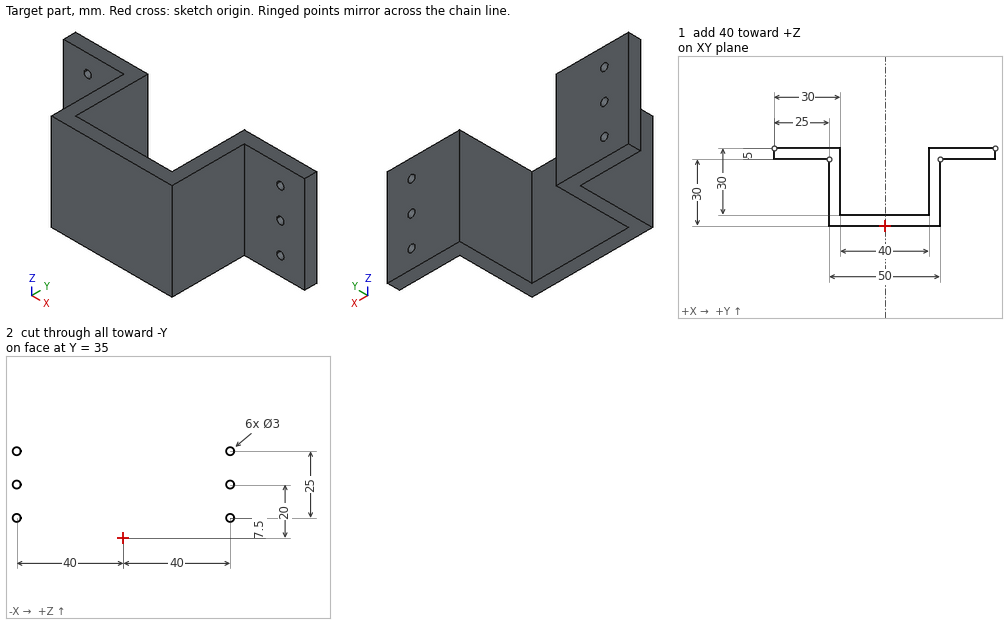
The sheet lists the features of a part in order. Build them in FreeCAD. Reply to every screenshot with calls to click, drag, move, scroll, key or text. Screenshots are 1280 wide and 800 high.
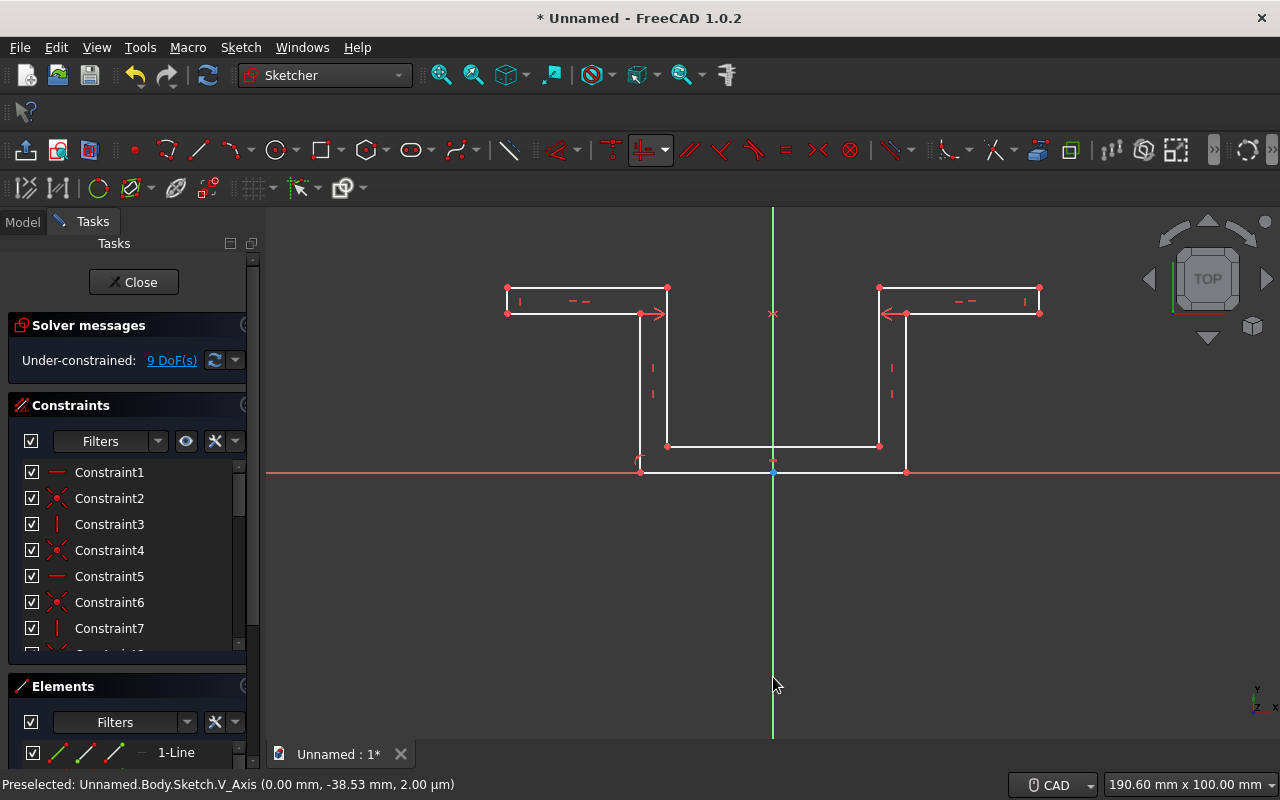
click(507, 288)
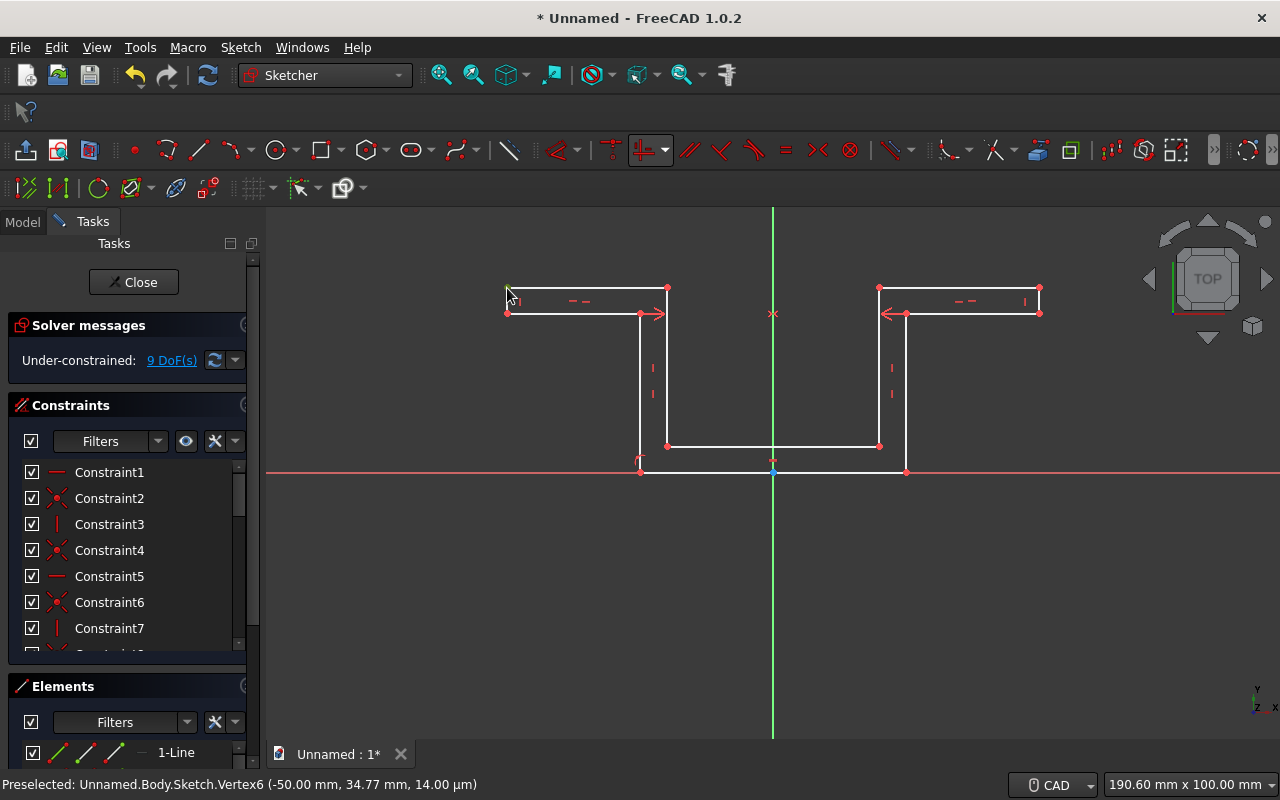
click(1039, 288)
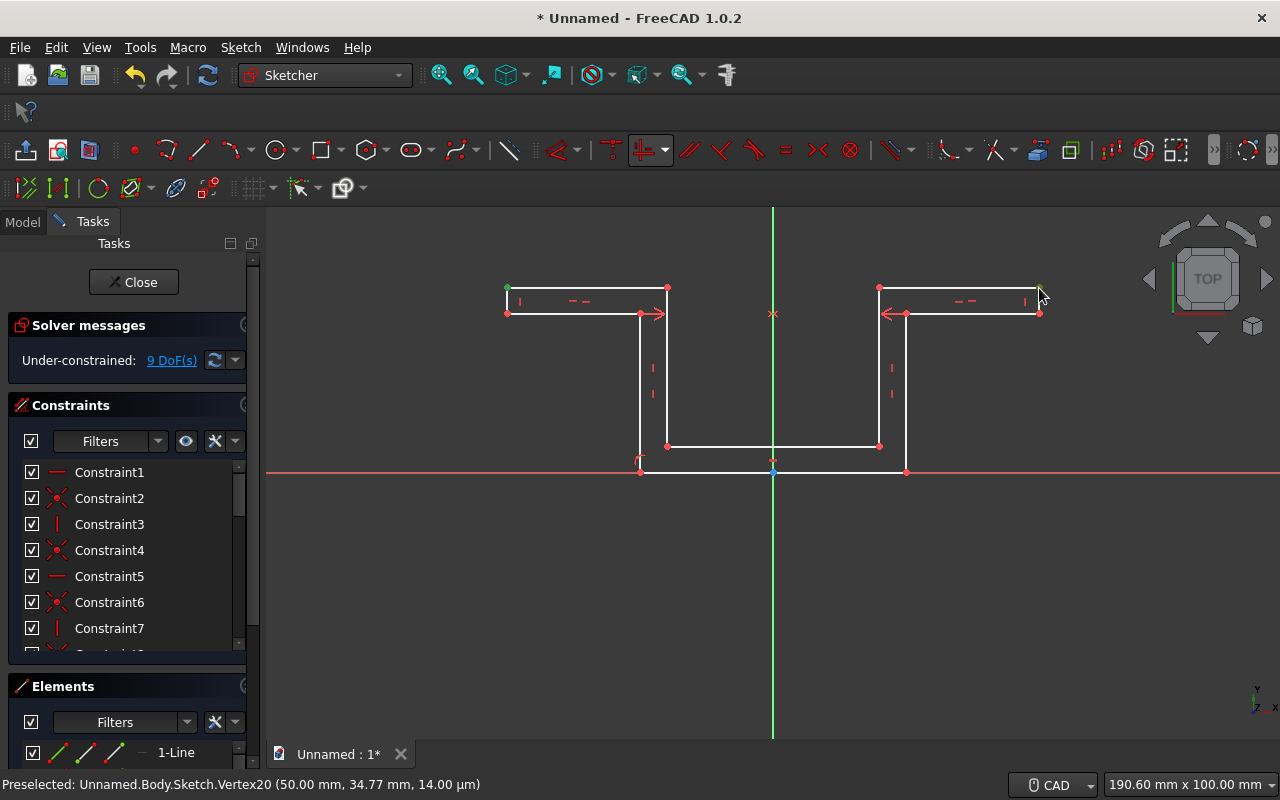
click(773, 677)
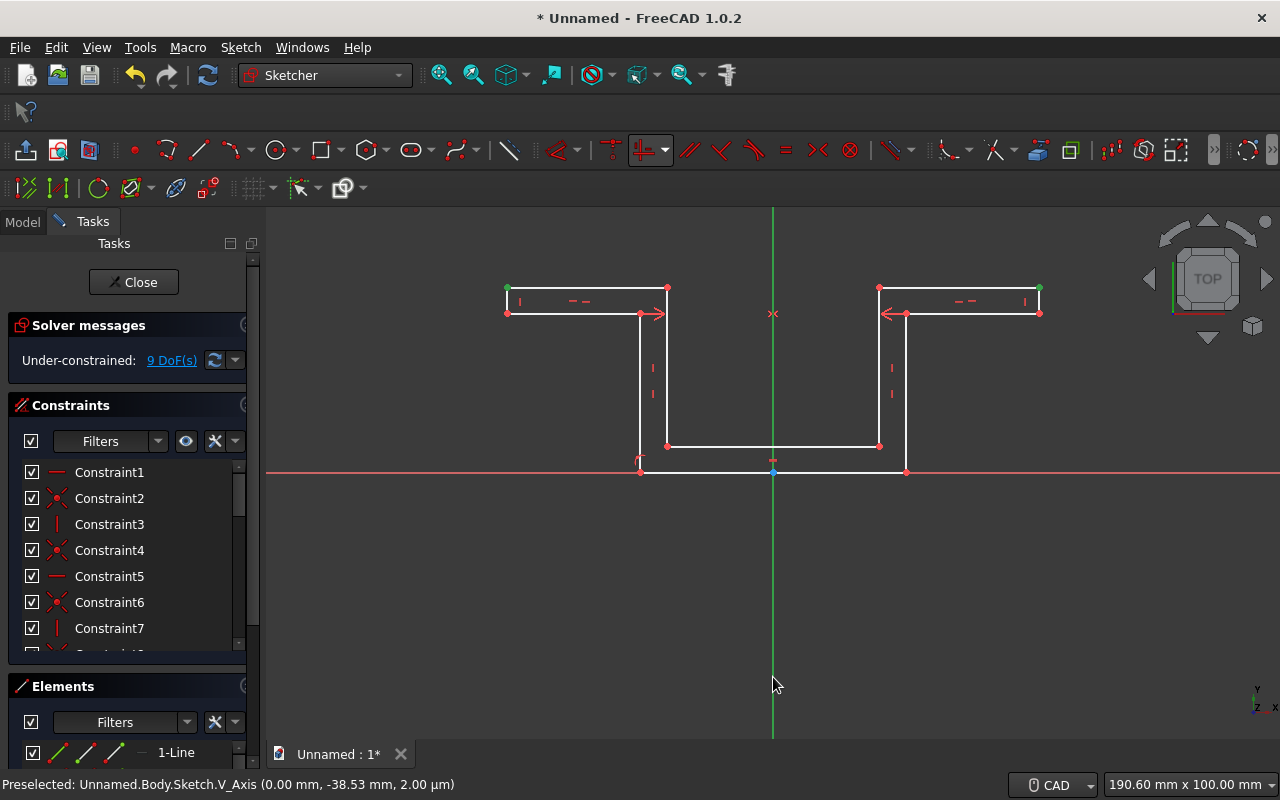
click(818, 150)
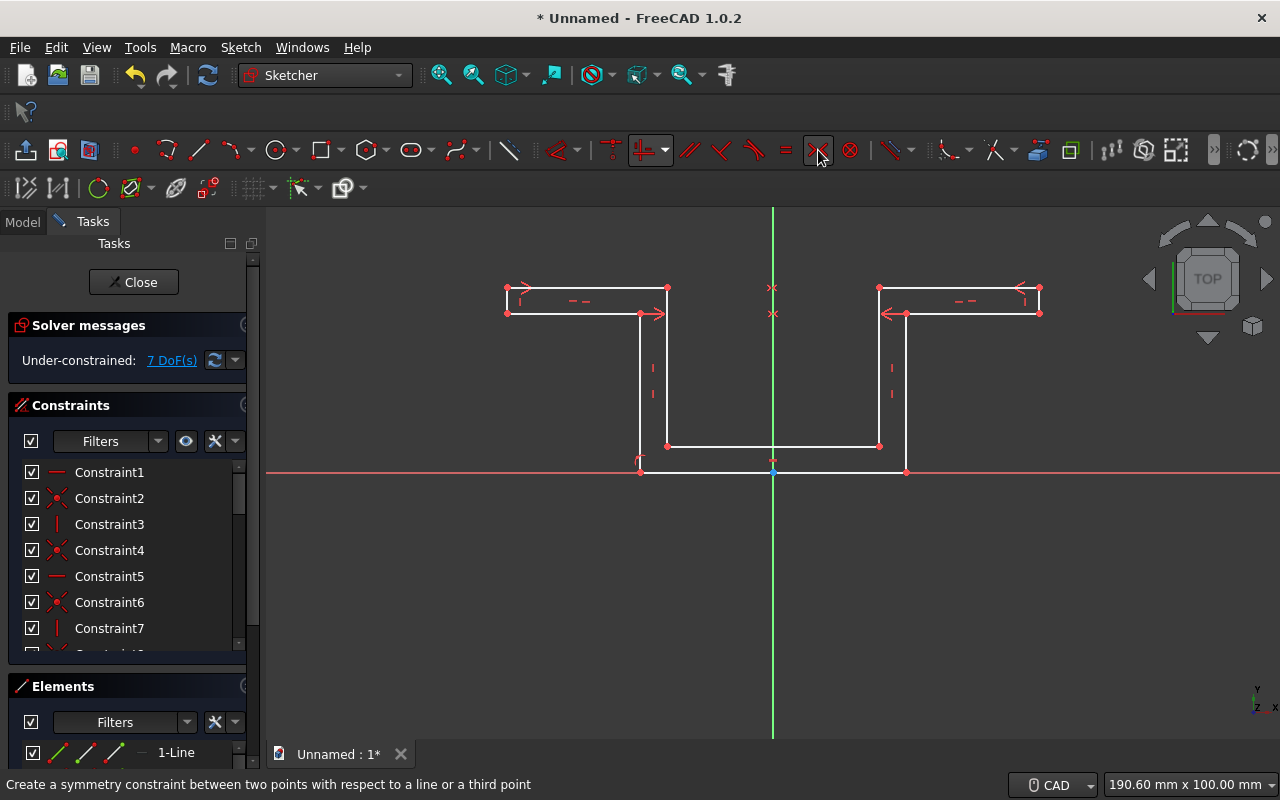
click(556, 150)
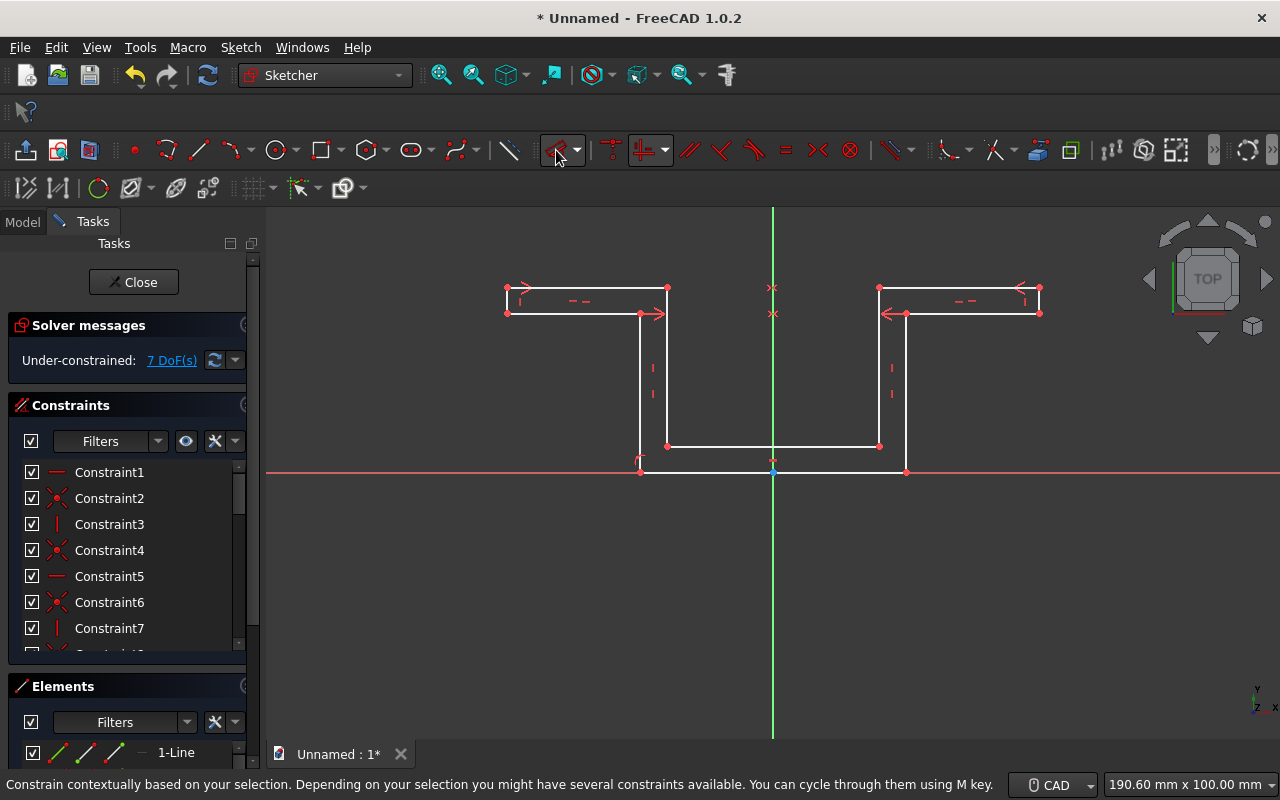
scroll(507, 298, up, 3)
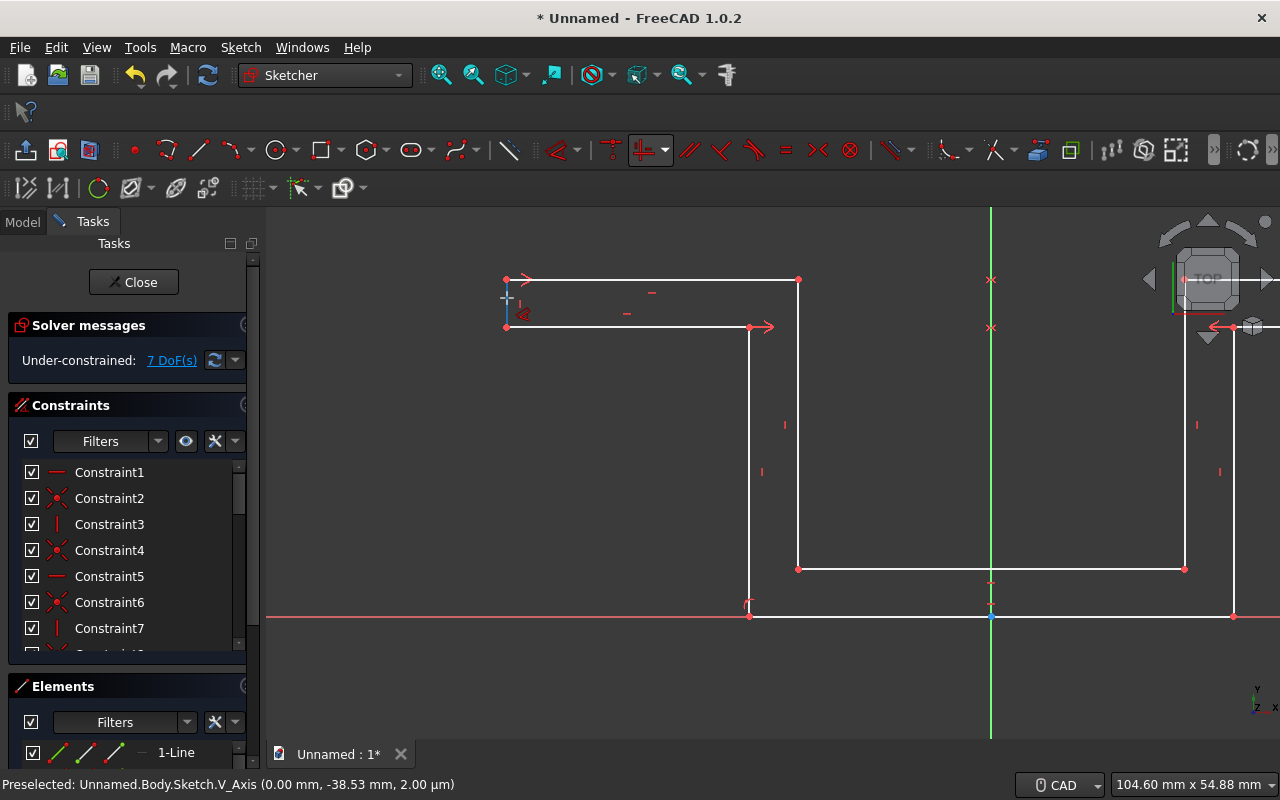
click(507, 299)
click(473, 303)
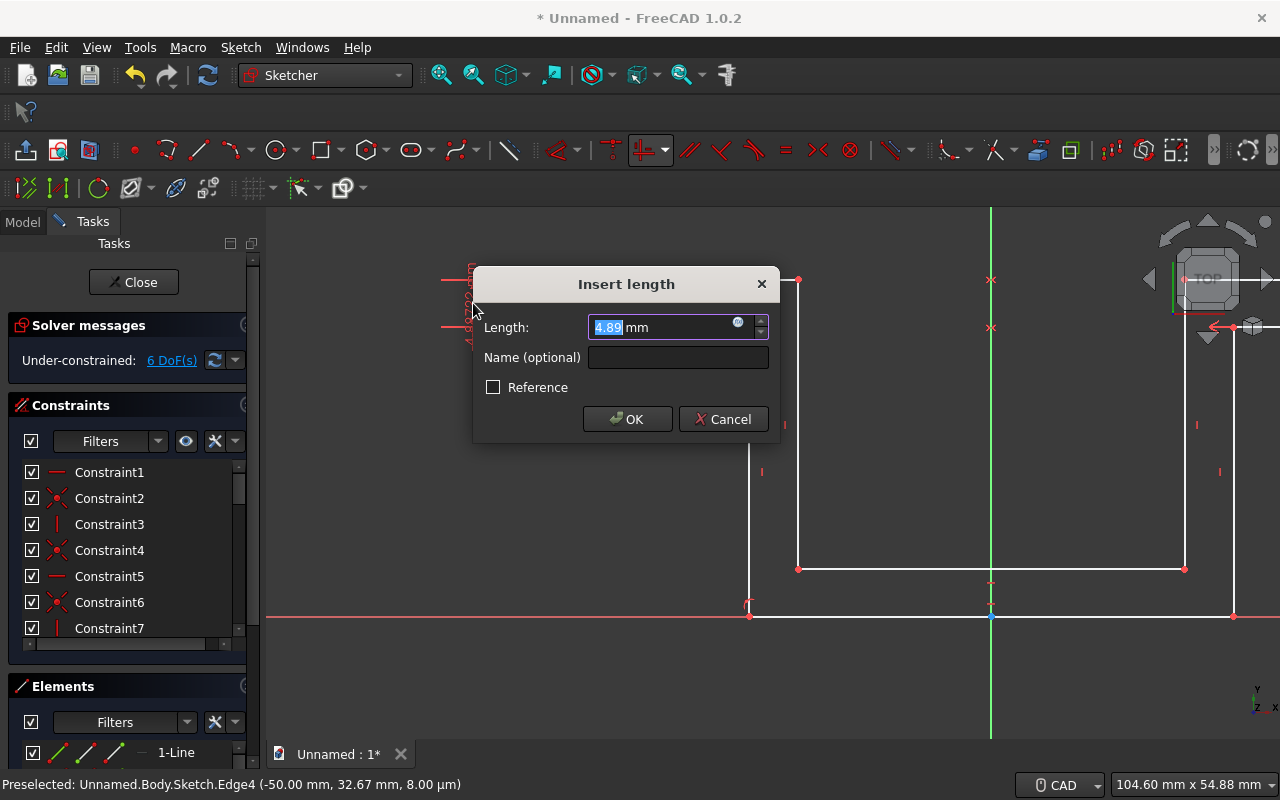
text(5)
key(Return)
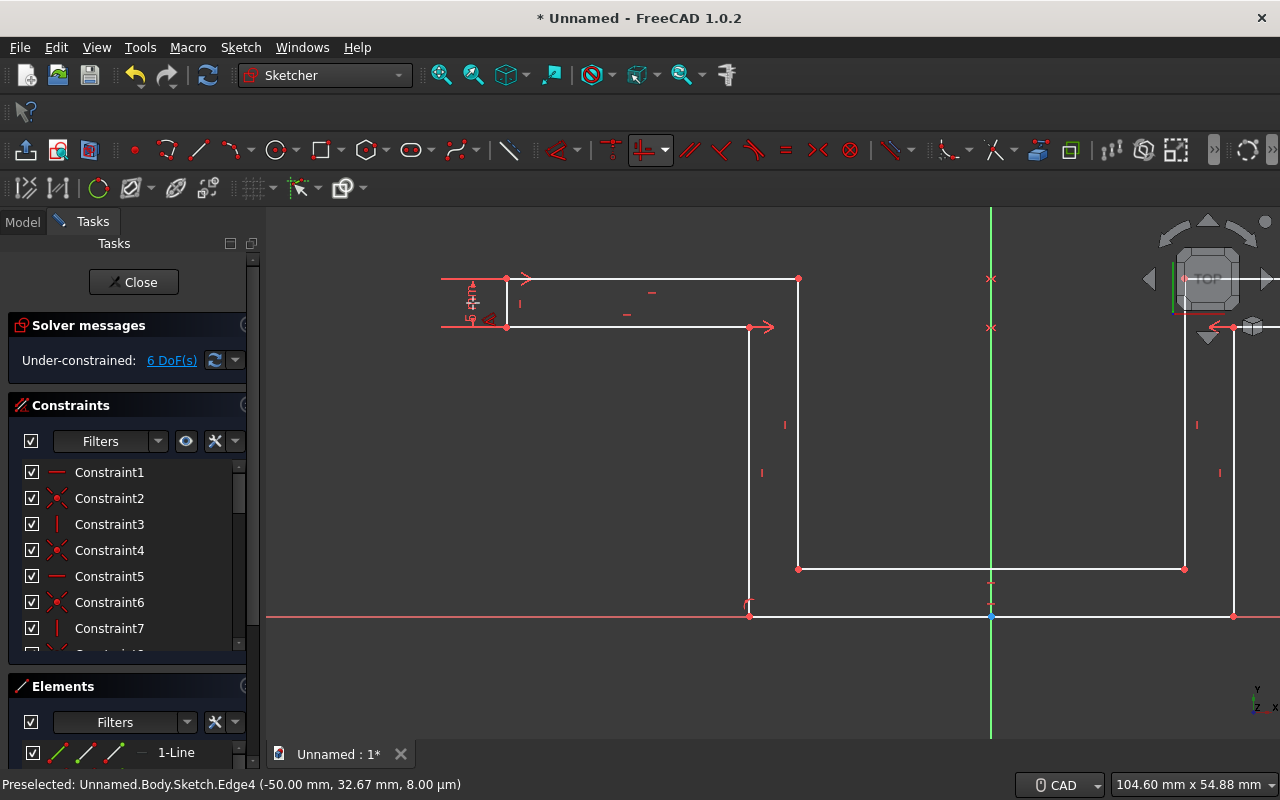
click(1069, 569)
click(957, 603)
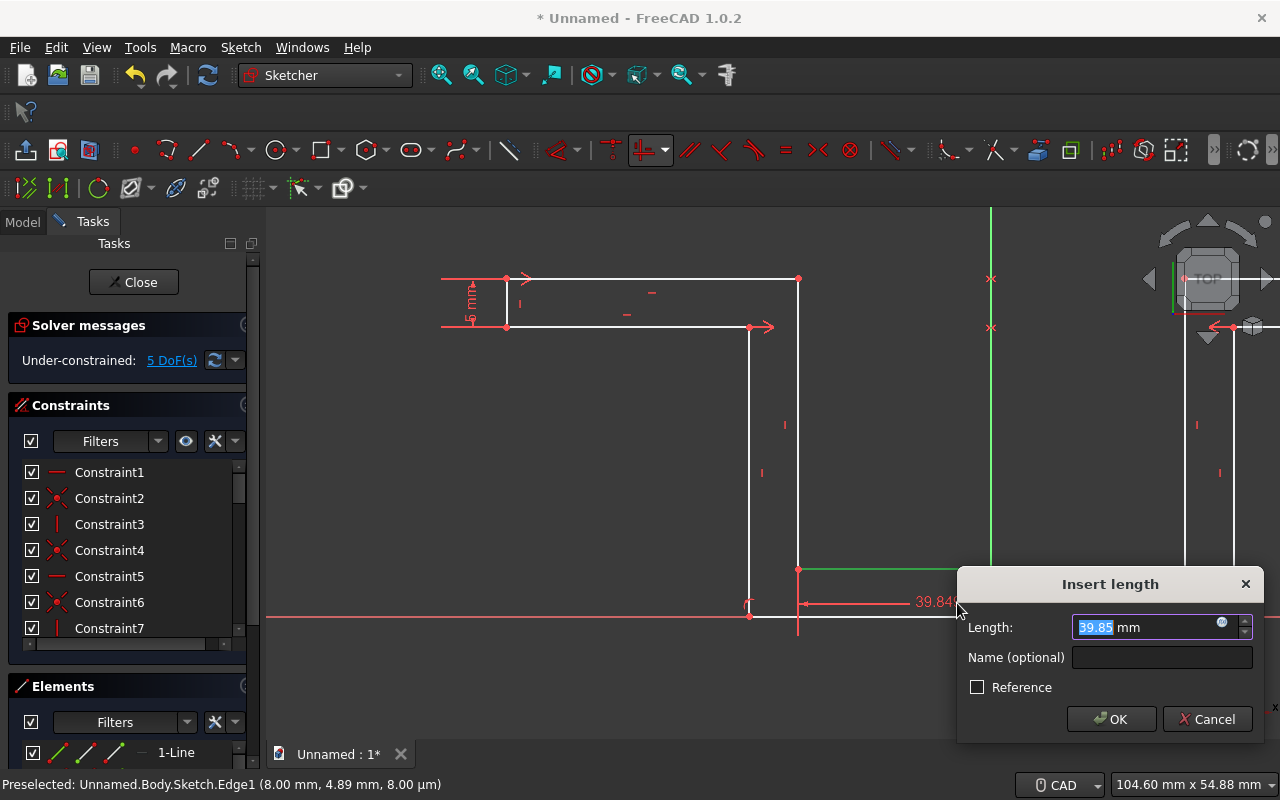
text(40)
key(Return)